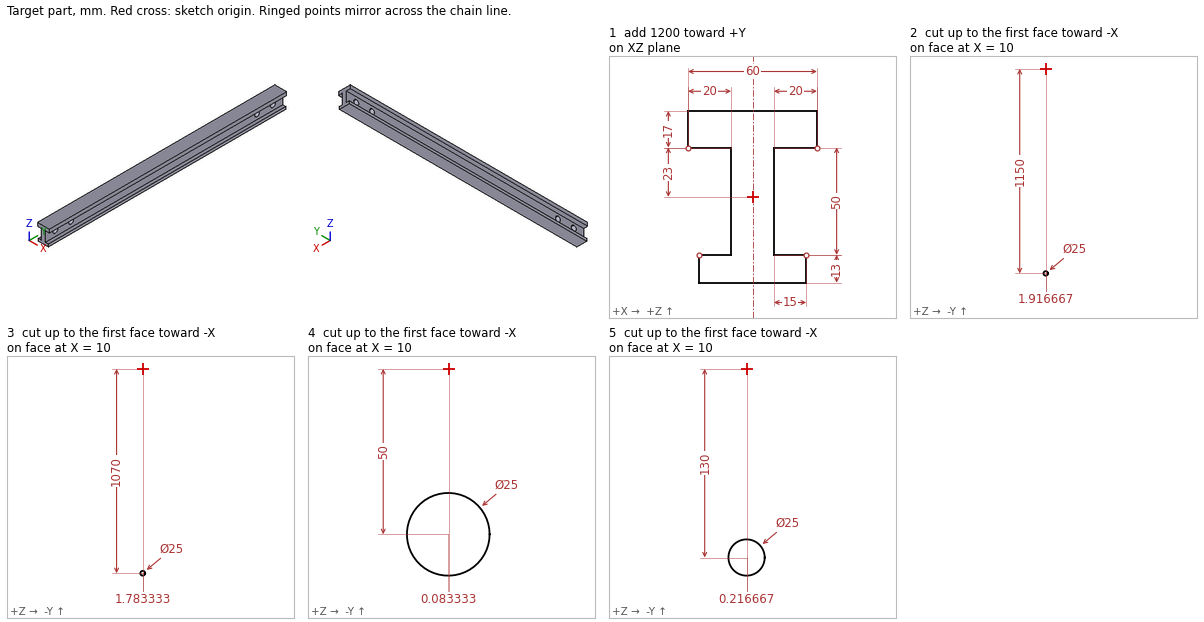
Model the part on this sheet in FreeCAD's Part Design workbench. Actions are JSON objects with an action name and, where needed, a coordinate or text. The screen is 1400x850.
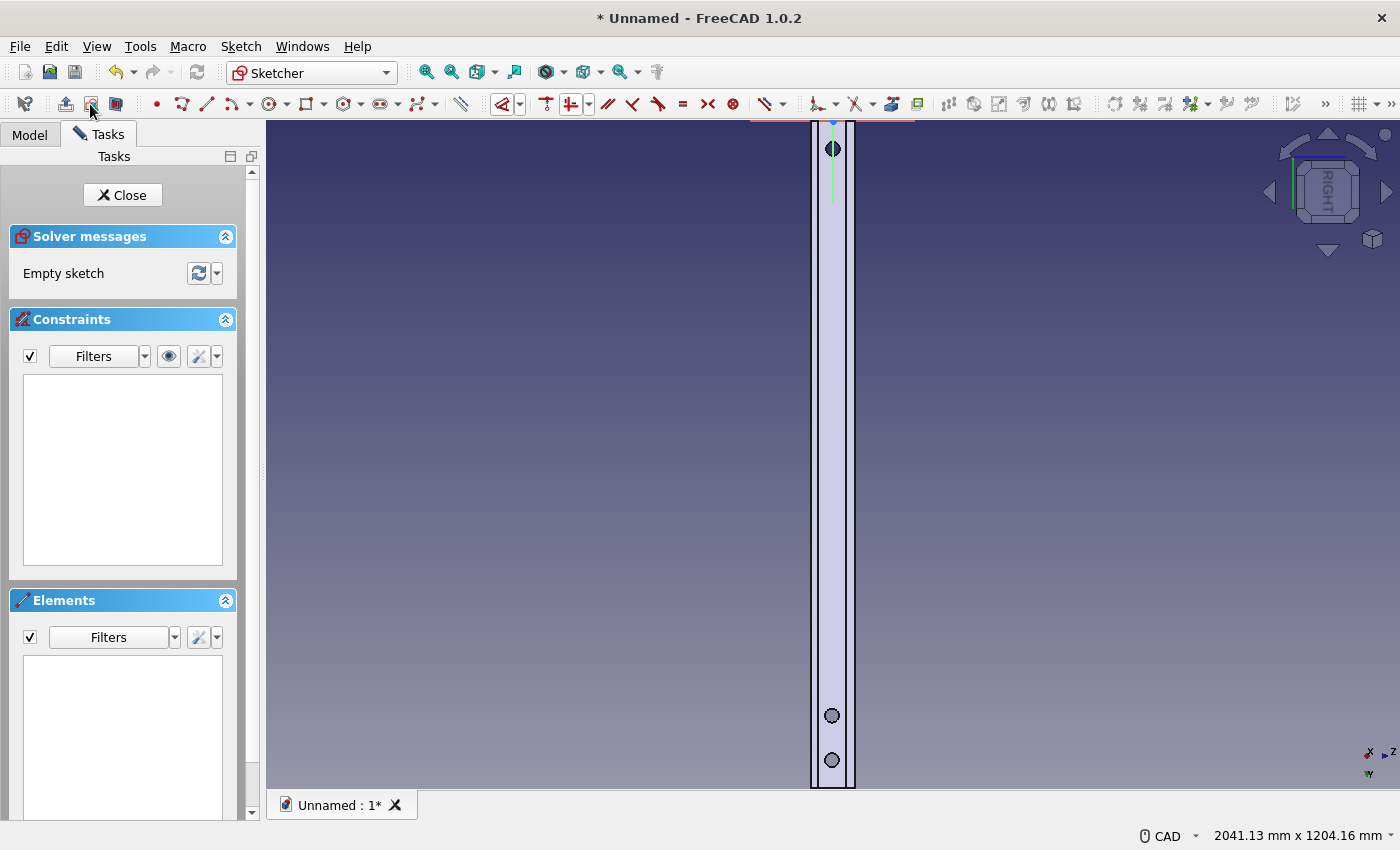
{"action": "scroll", "coordinate": [836, 180], "scroll_direction": "up", "scroll_amount": 15}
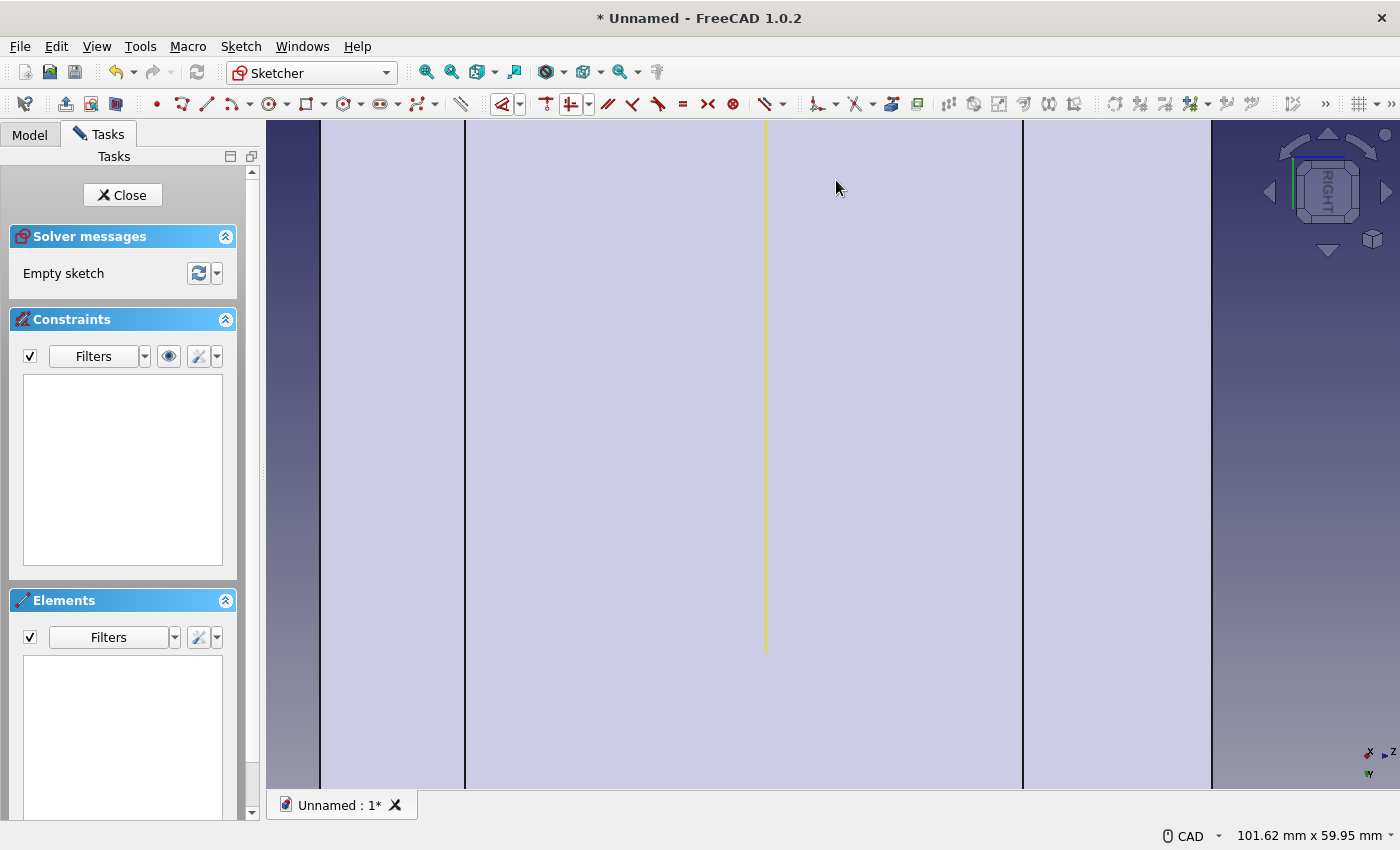
{"action": "scroll", "coordinate": [762, 432], "scroll_direction": "up", "scroll_amount": 2}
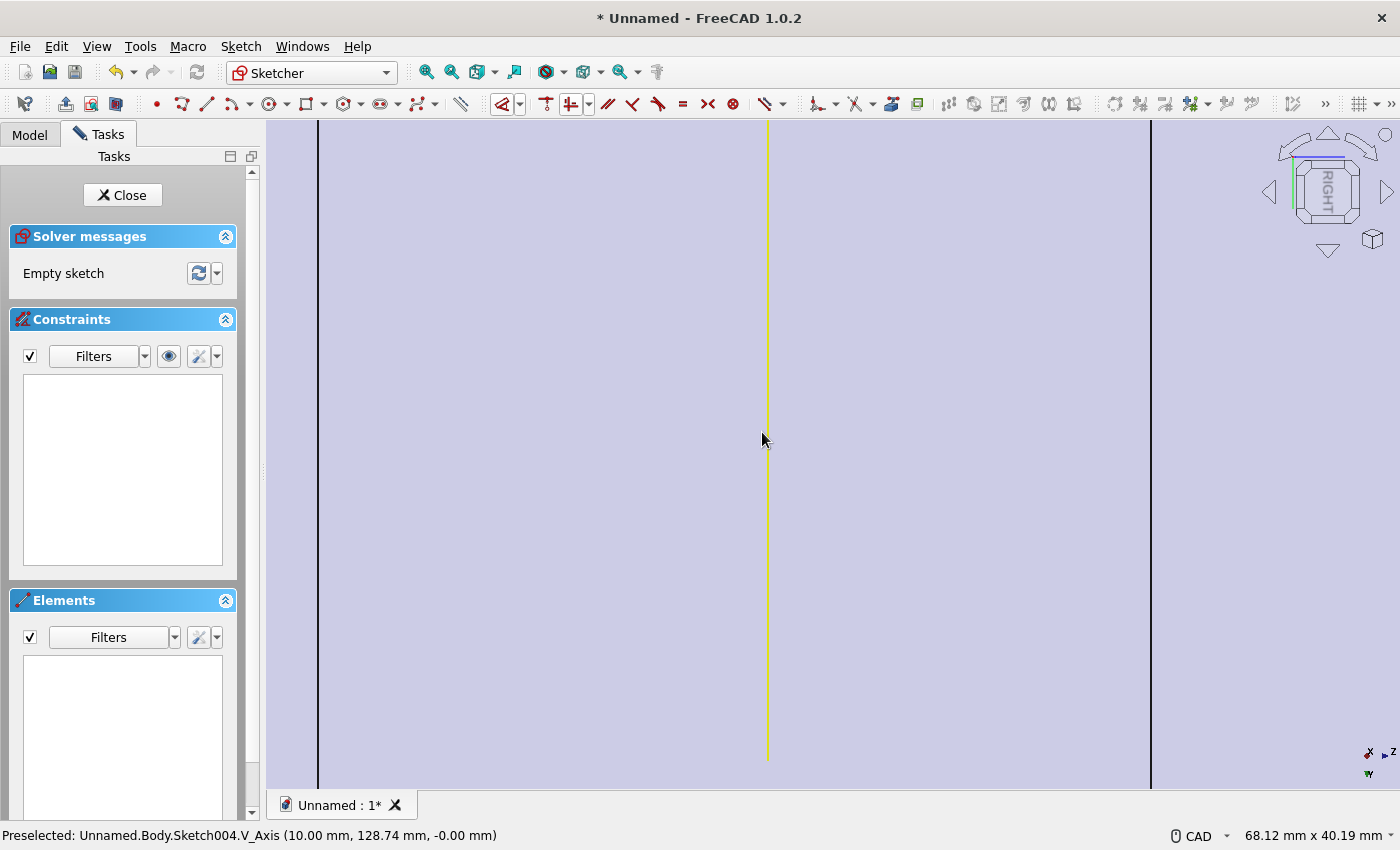
{"action": "left_click", "coordinate": [268, 104]}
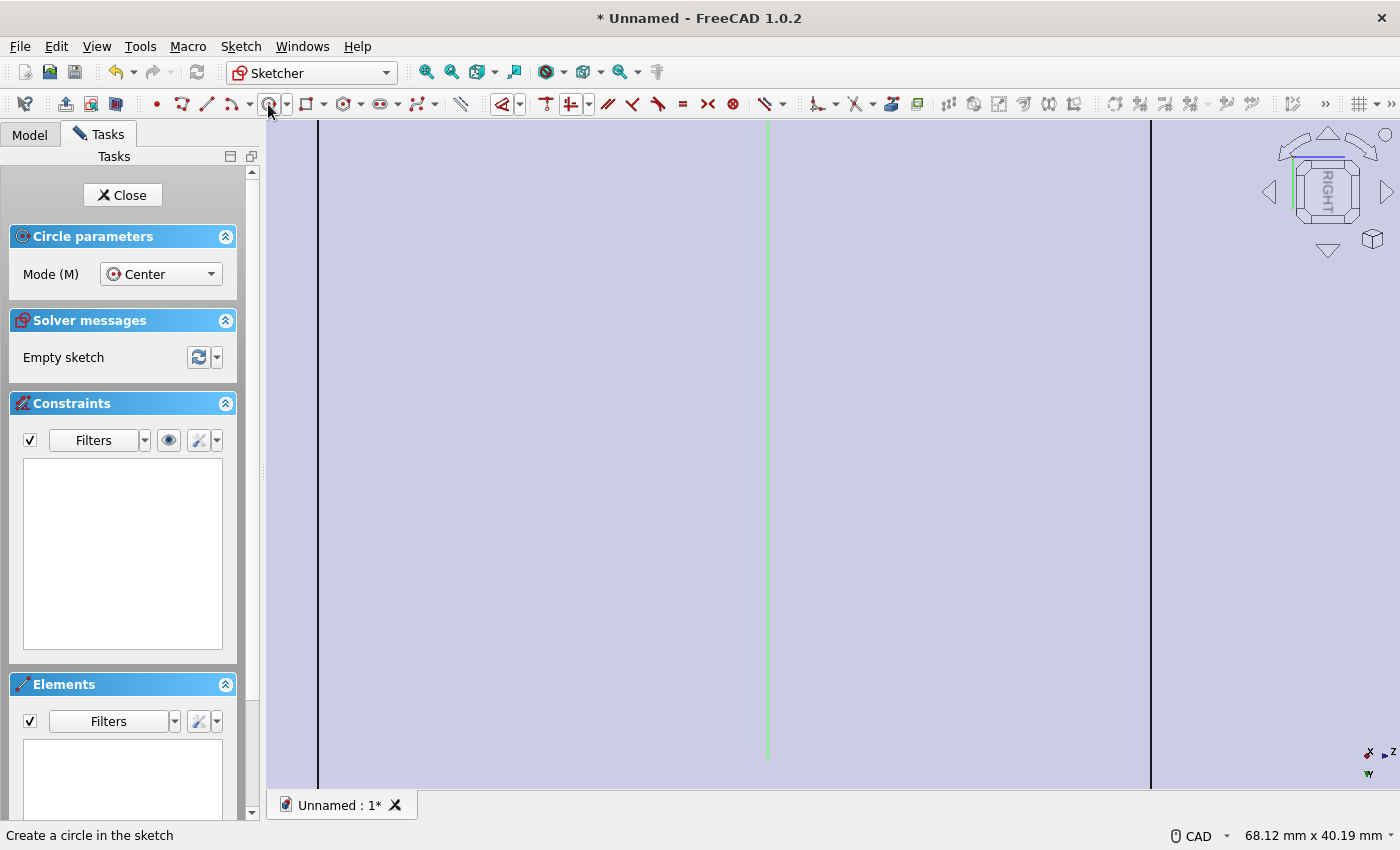
{"action": "scroll", "coordinate": [764, 454], "scroll_direction": "up", "scroll_amount": 8}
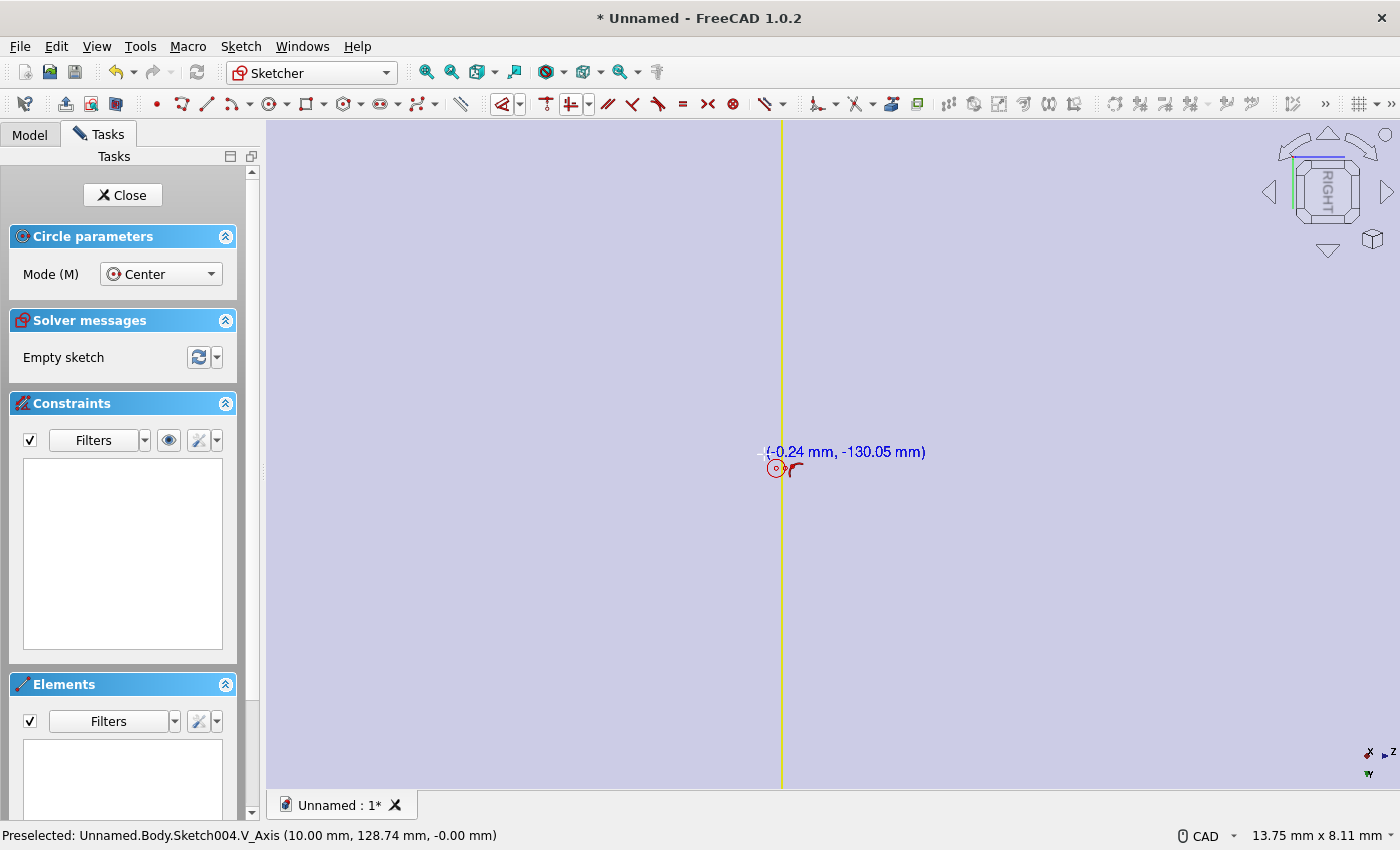
{"action": "left_click", "coordinate": [764, 453]}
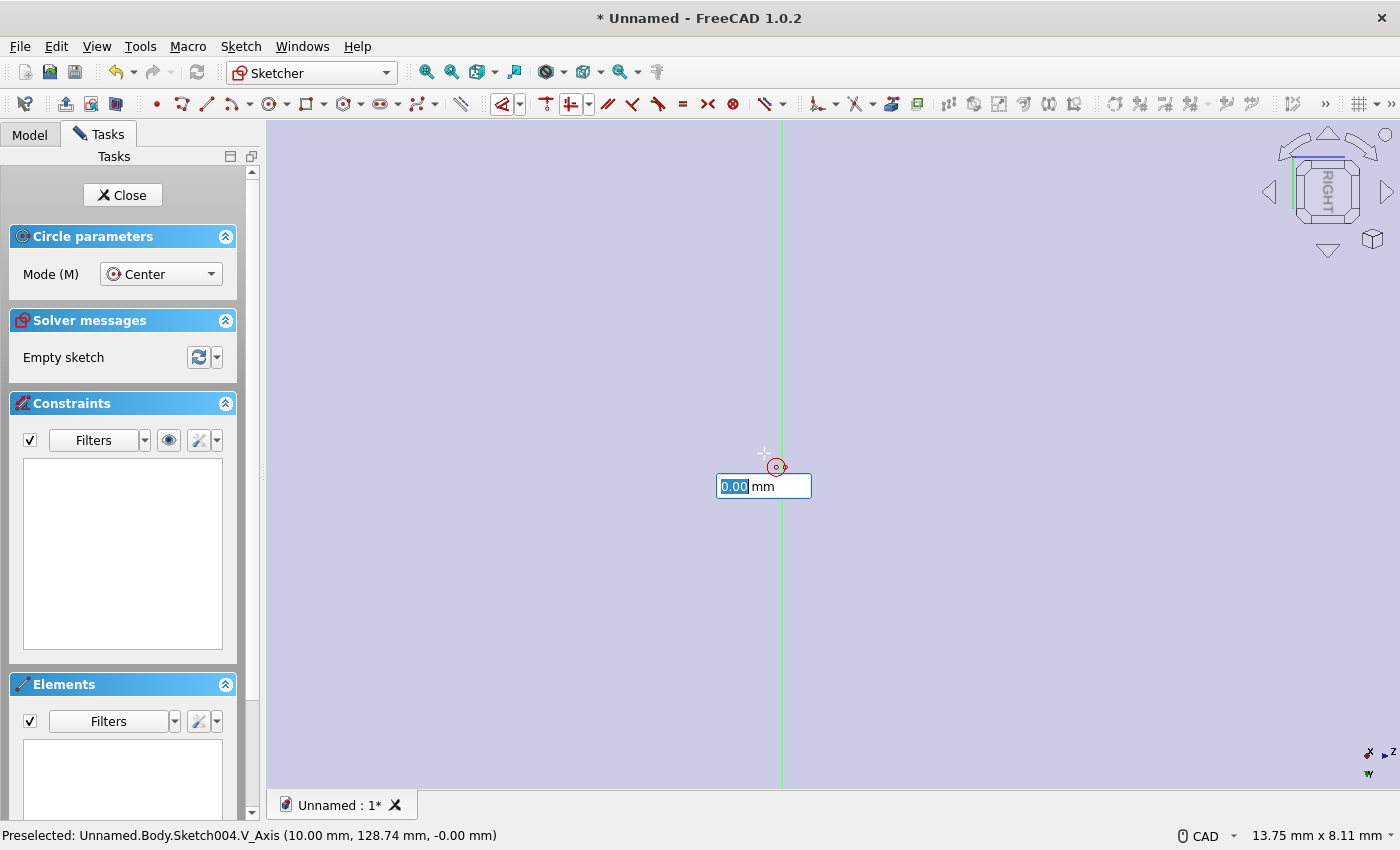
{"action": "scroll", "coordinate": [765, 455], "scroll_direction": "down", "scroll_amount": 8}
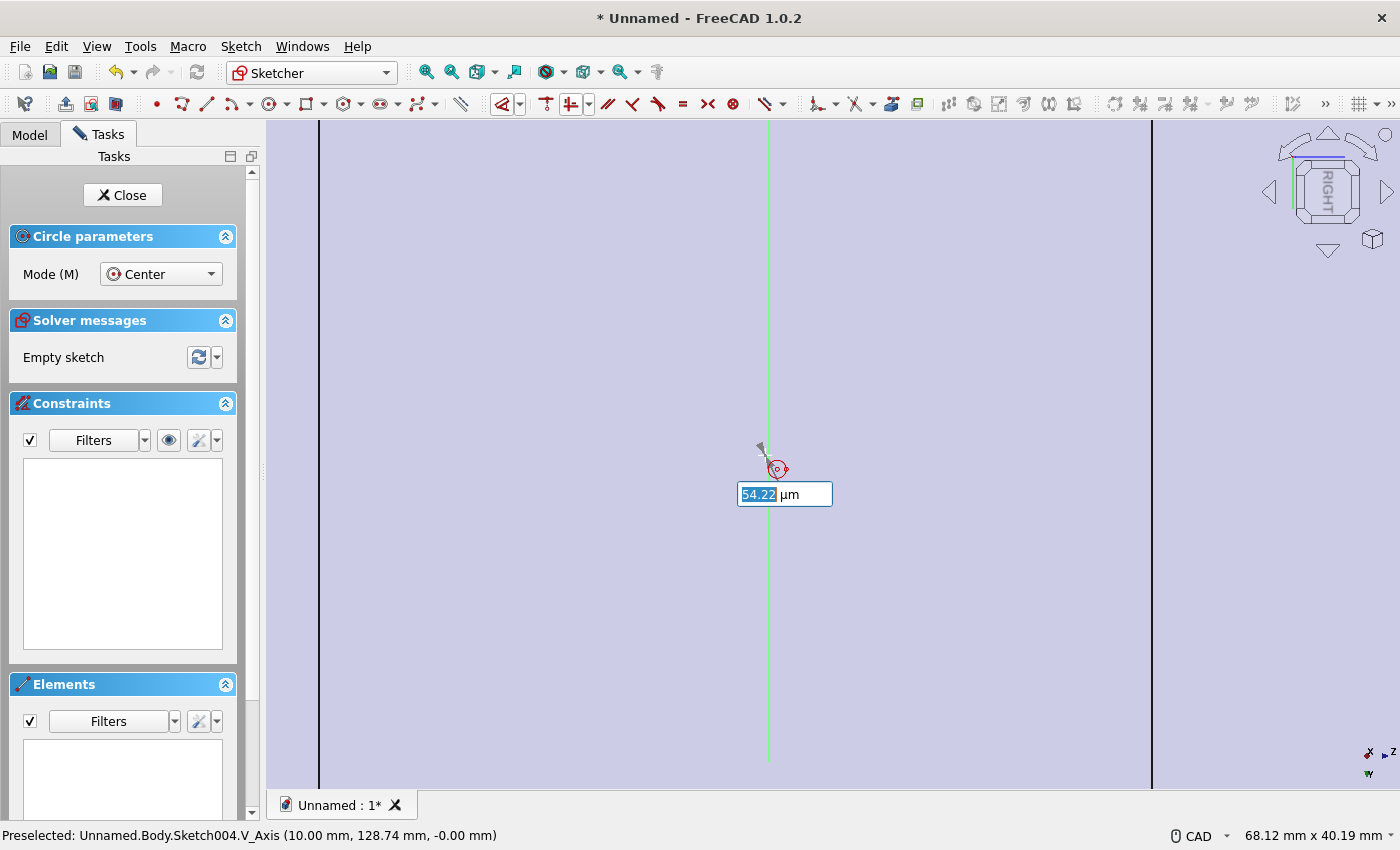
{"action": "left_click", "coordinate": [912, 308]}
{"action": "key", "text": "Escape"}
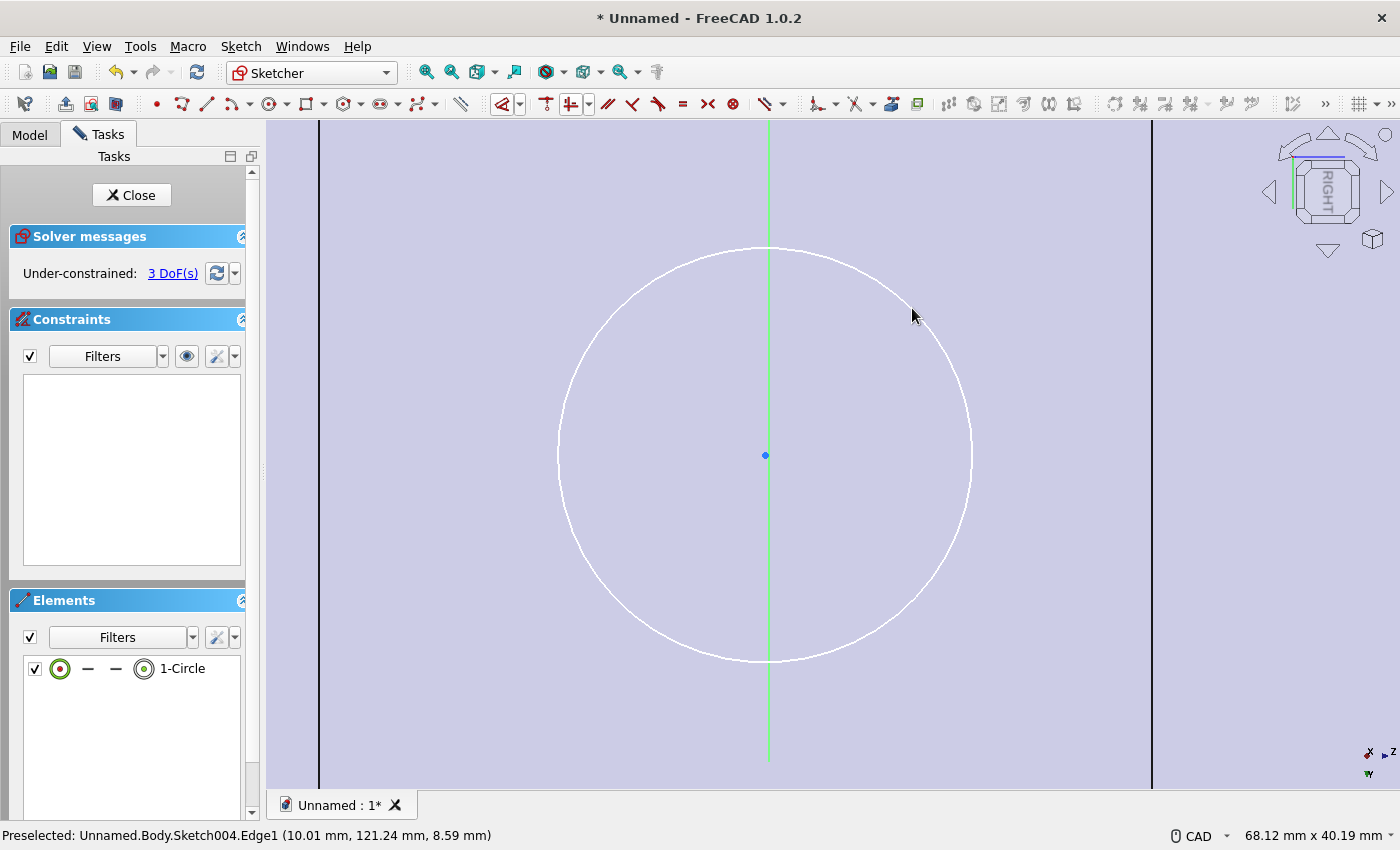
{"action": "left_click", "coordinate": [911, 308]}